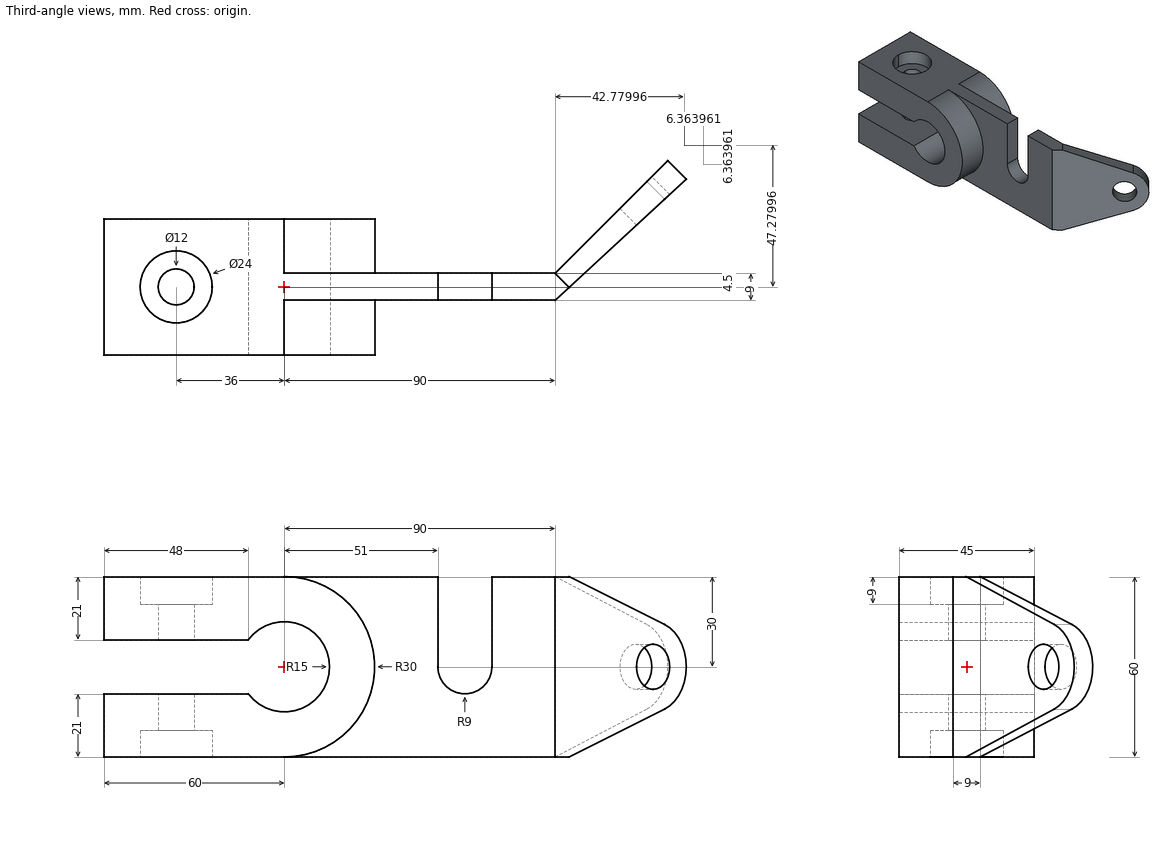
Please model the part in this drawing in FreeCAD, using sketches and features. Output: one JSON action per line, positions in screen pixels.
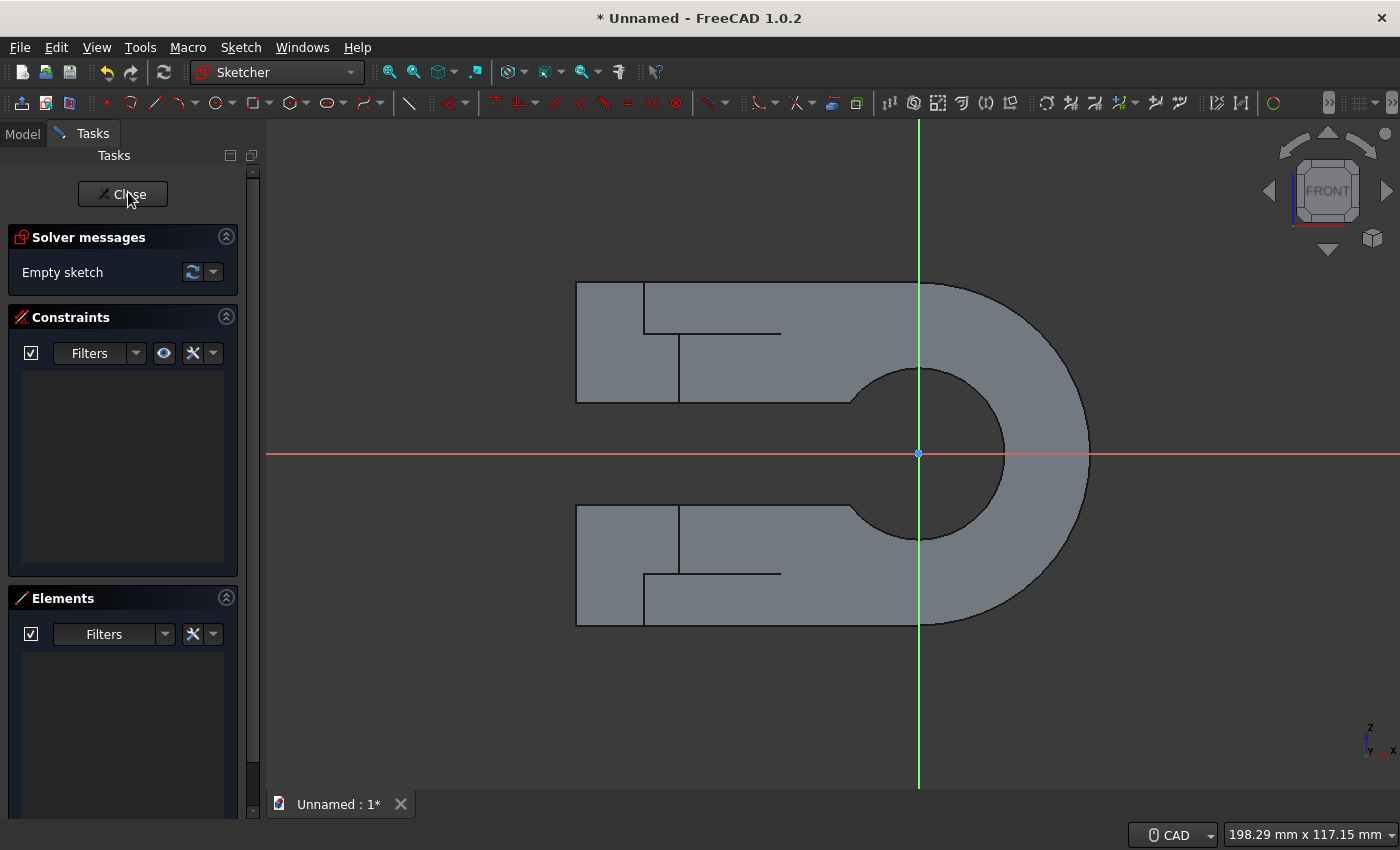
{"action": "scroll", "coordinate": [294, 454], "scroll_direction": "down", "scroll_amount": 2}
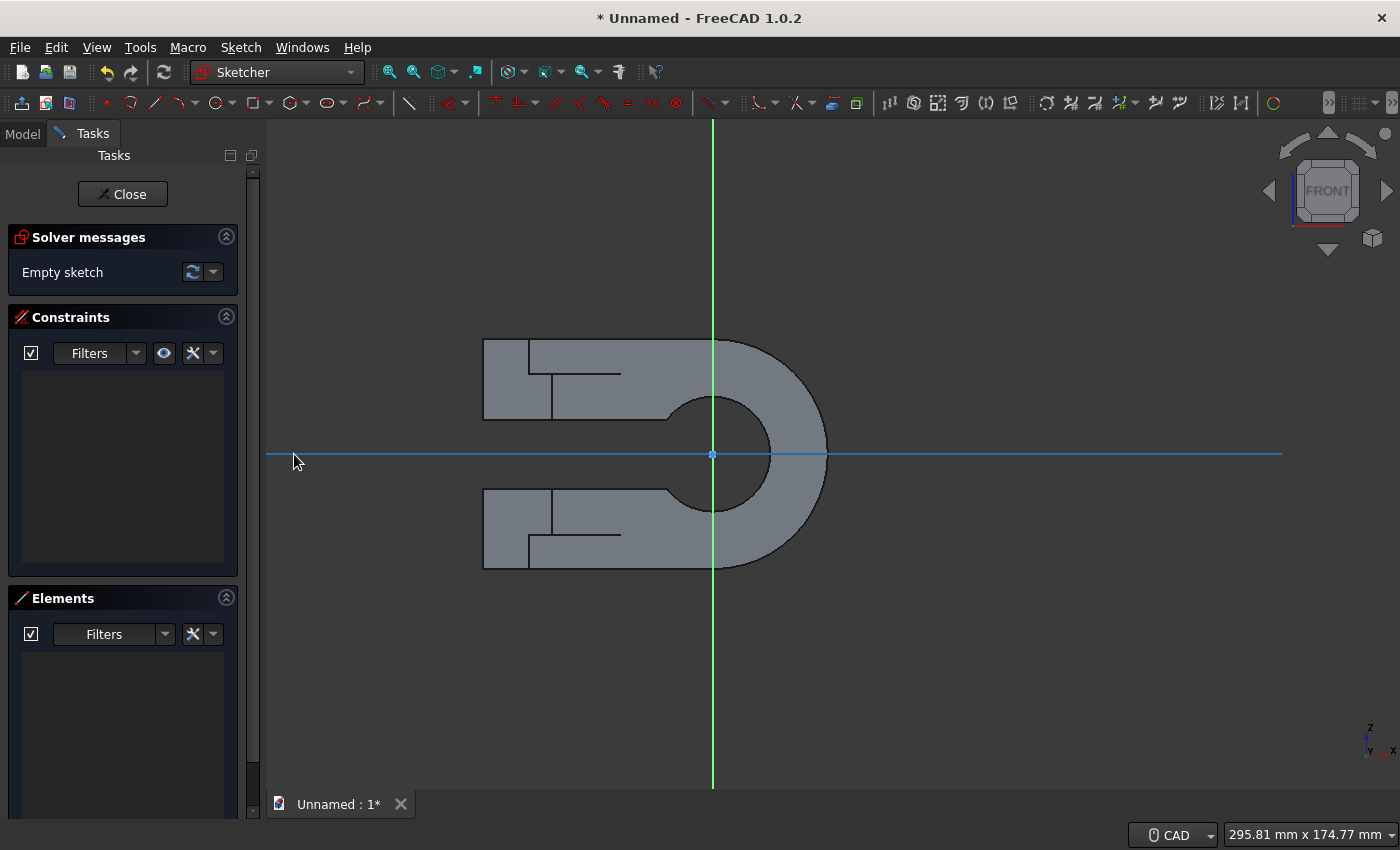
{"action": "scroll", "coordinate": [1032, 454], "scroll_direction": "up", "scroll_amount": 3}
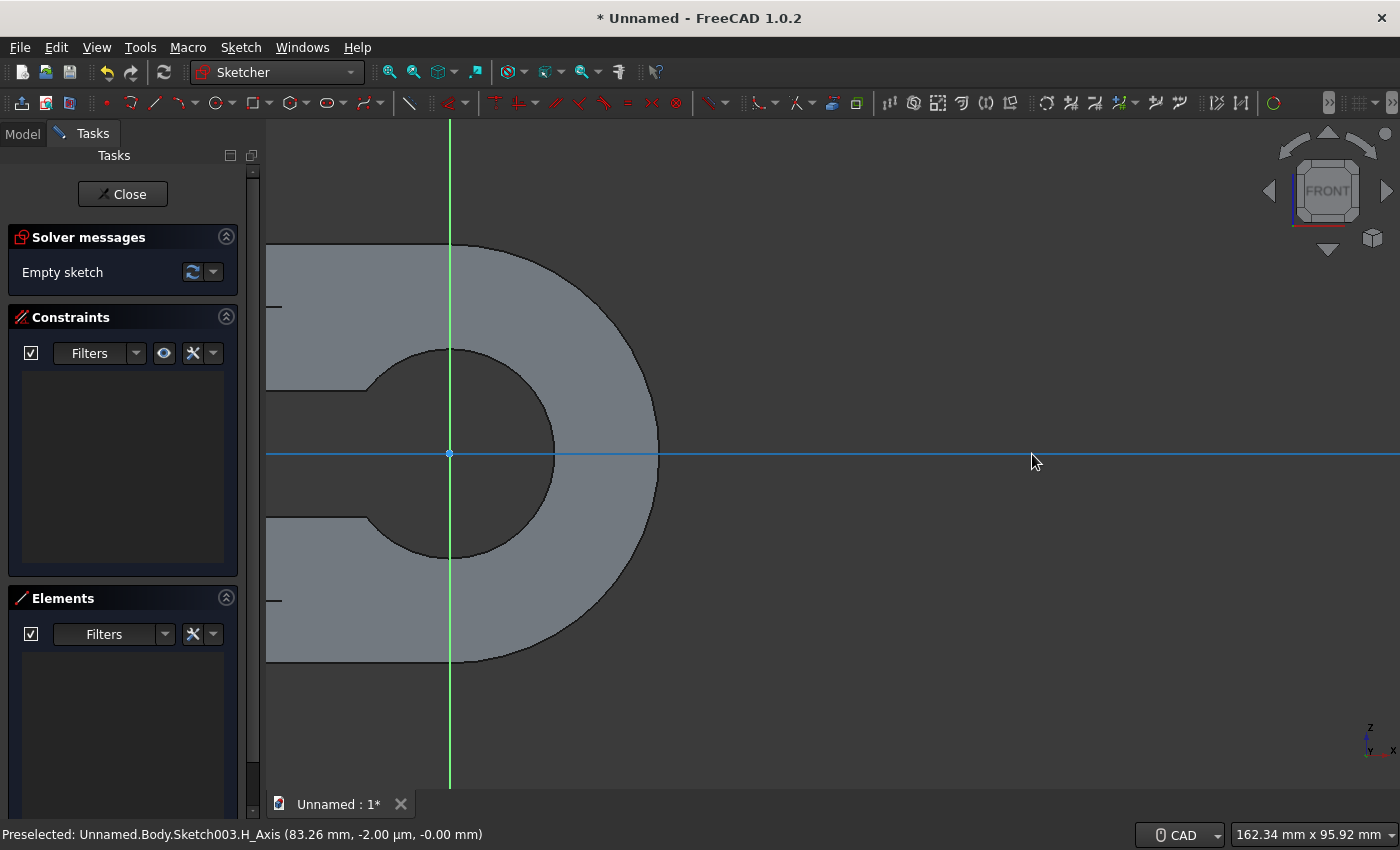
{"action": "key", "text": "g m"}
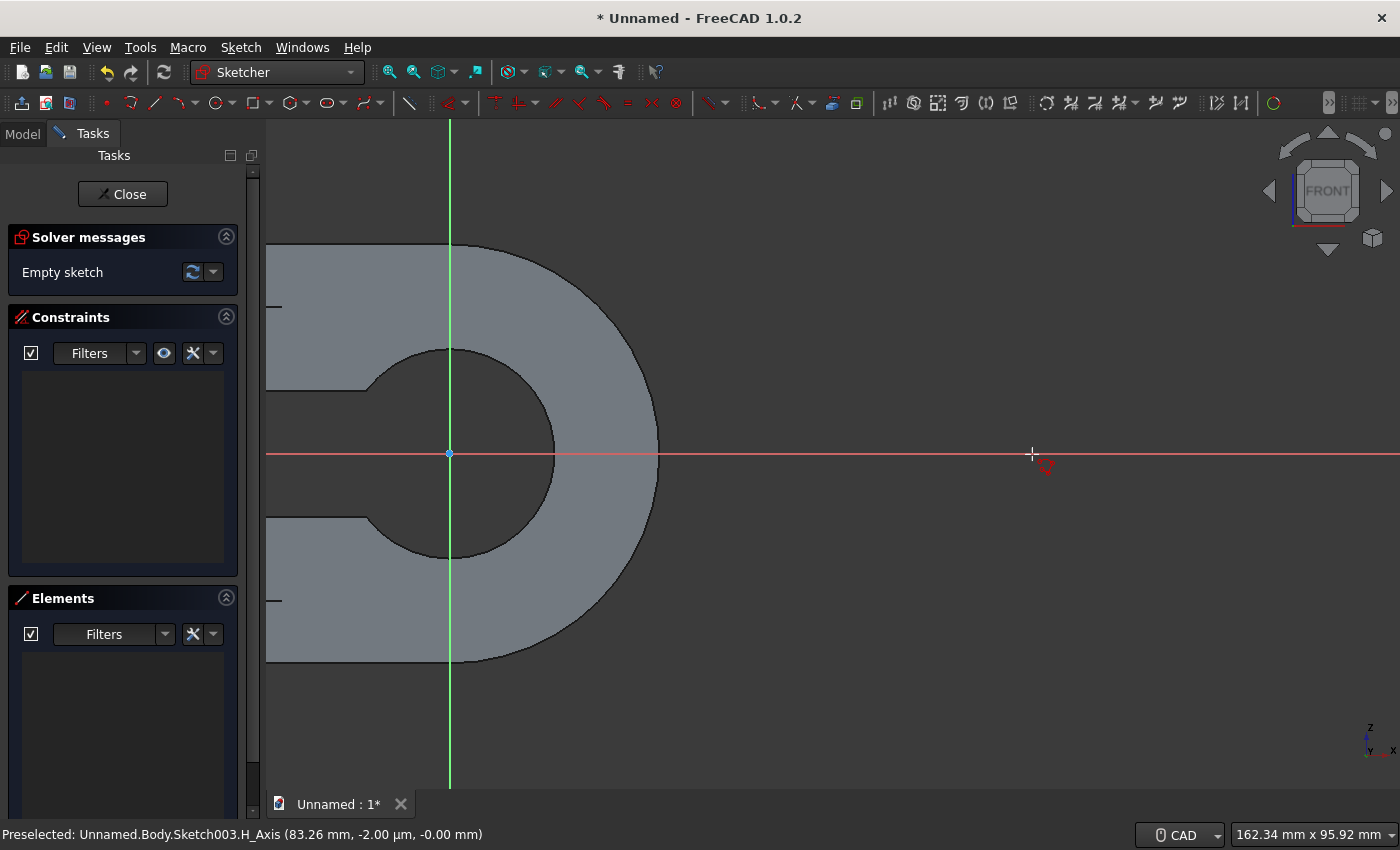
{"action": "left_click", "coordinate": [450, 244]}
{"action": "left_click", "coordinate": [1079, 244]}
{"action": "left_click", "coordinate": [1079, 663]}
{"action": "left_click", "coordinate": [450, 663]}
{"action": "right_click", "coordinate": [450, 663]}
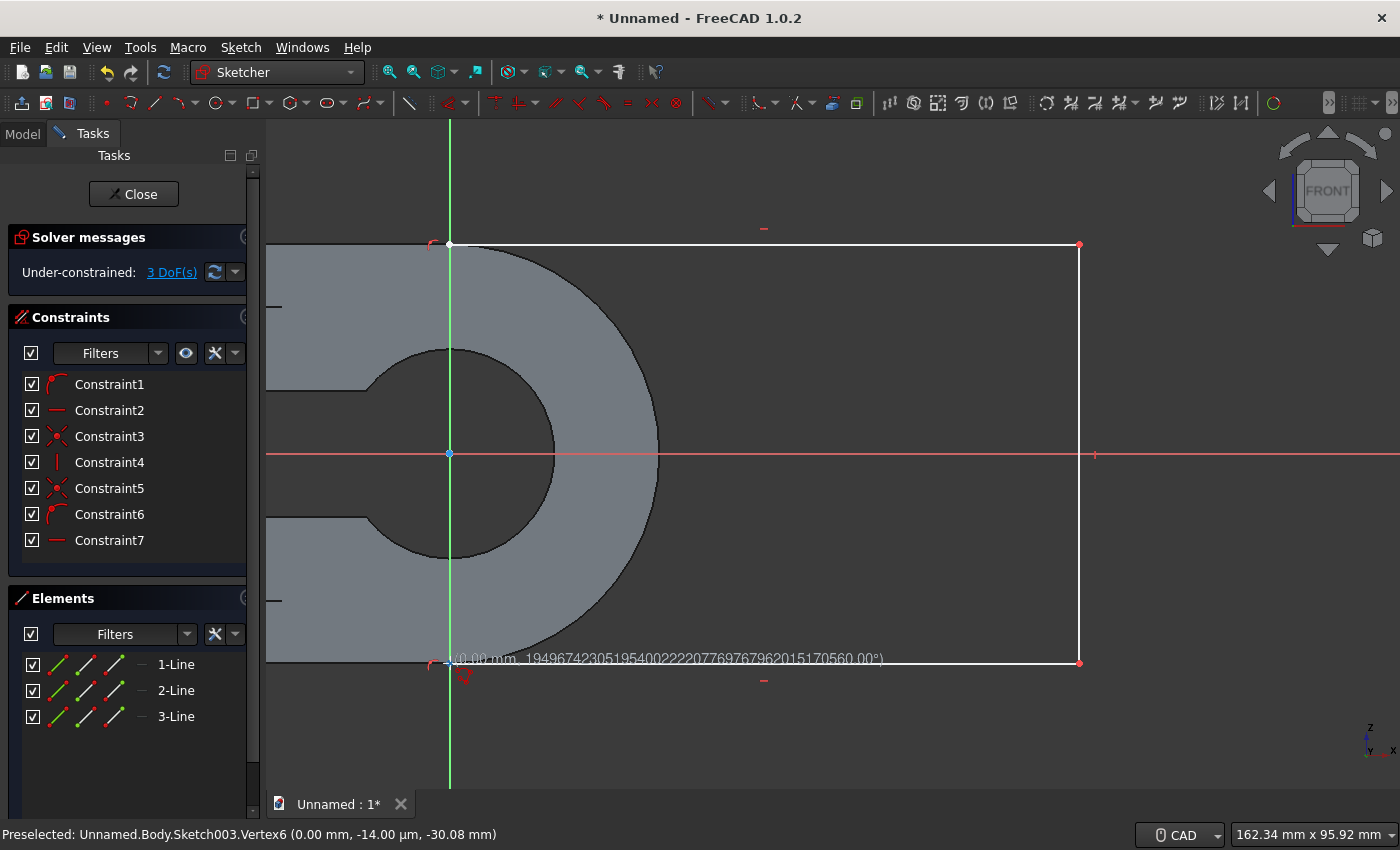
{"action": "key", "text": "g 3 a"}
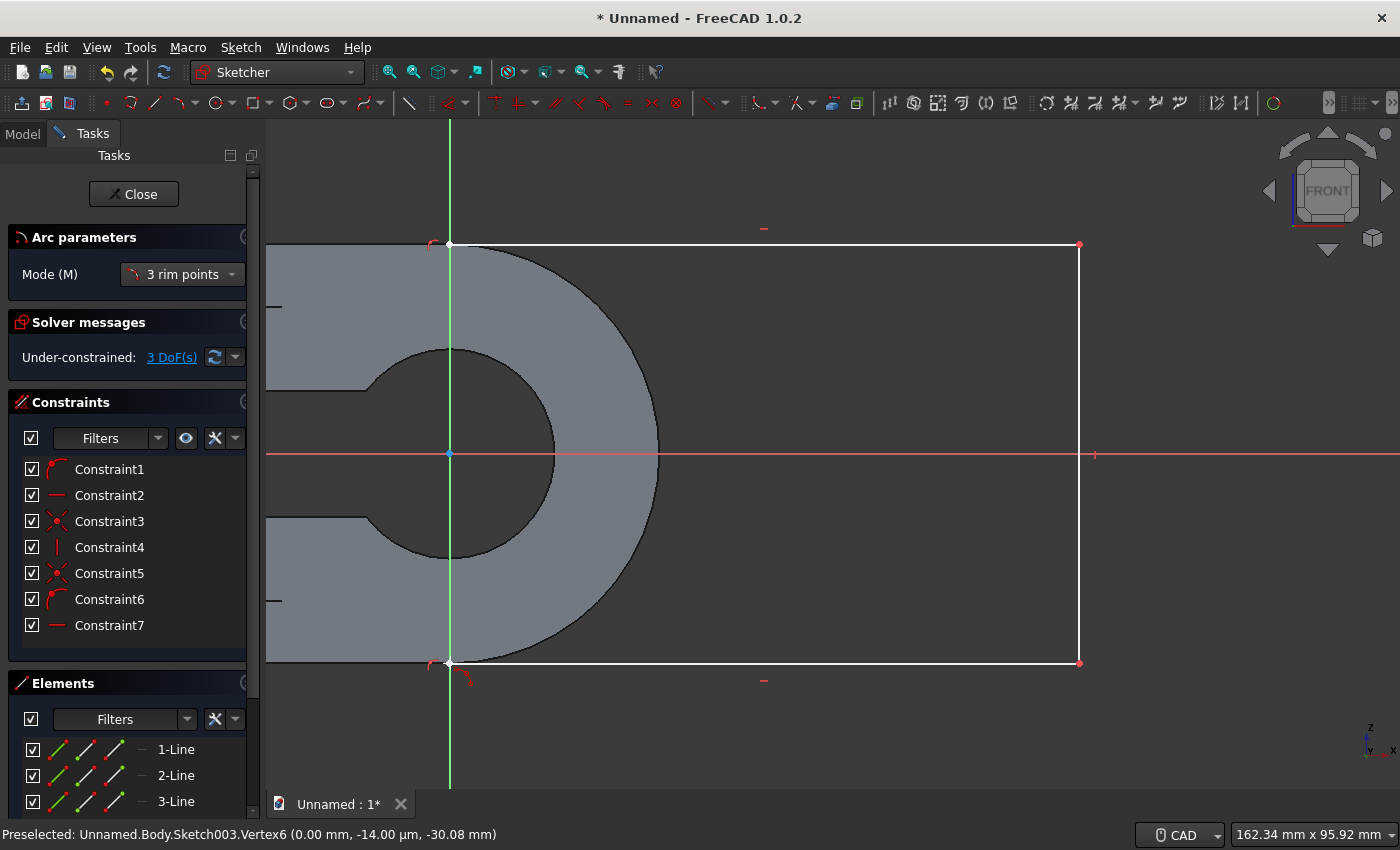
{"action": "left_click", "coordinate": [450, 664]}
{"action": "left_click", "coordinate": [450, 245]}
{"action": "left_click", "coordinate": [649, 519]}
{"action": "key", "text": "Escape"}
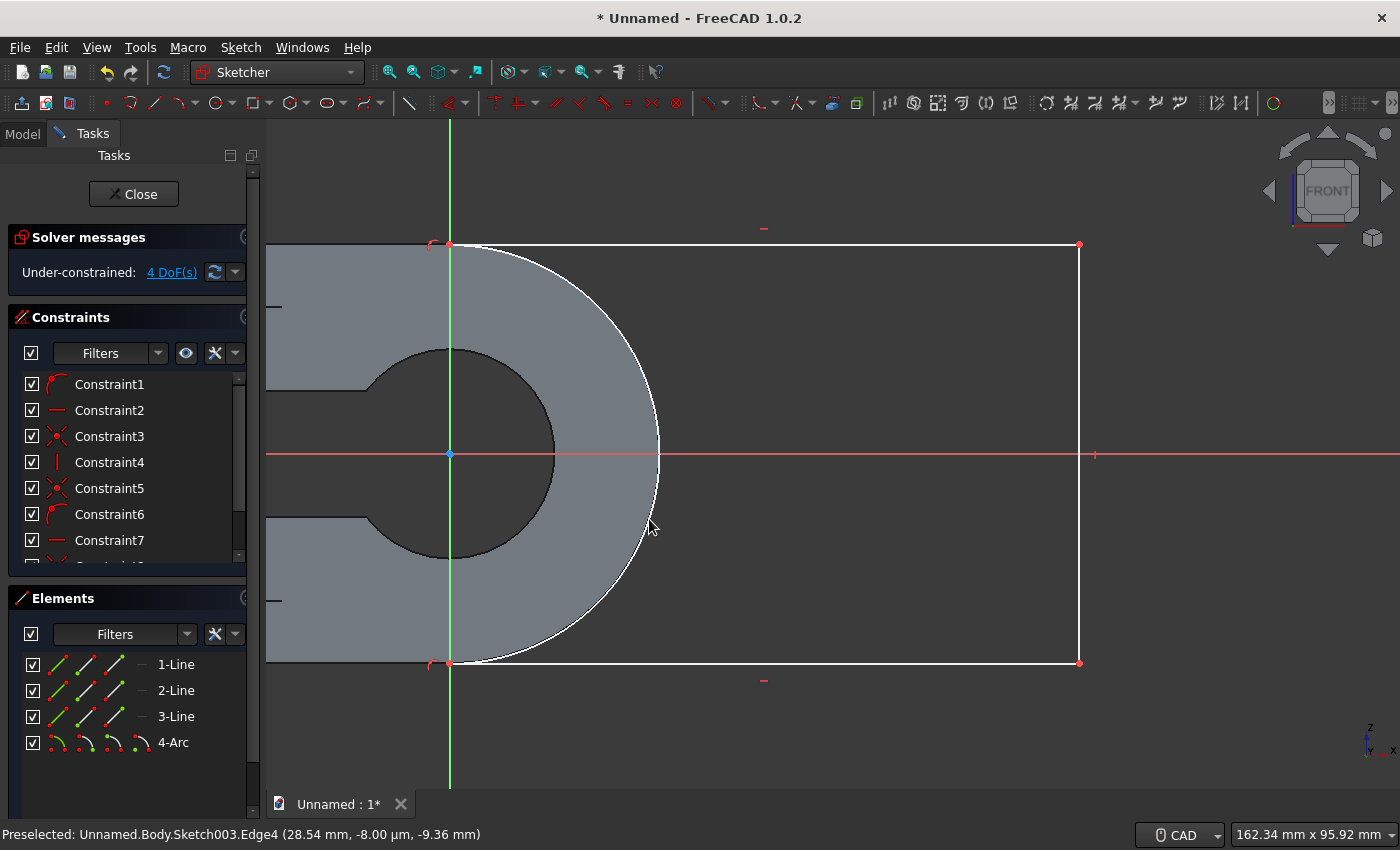
{"action": "left_click_drag", "start_coordinate": [440, 444], "coordinate": [460, 464]}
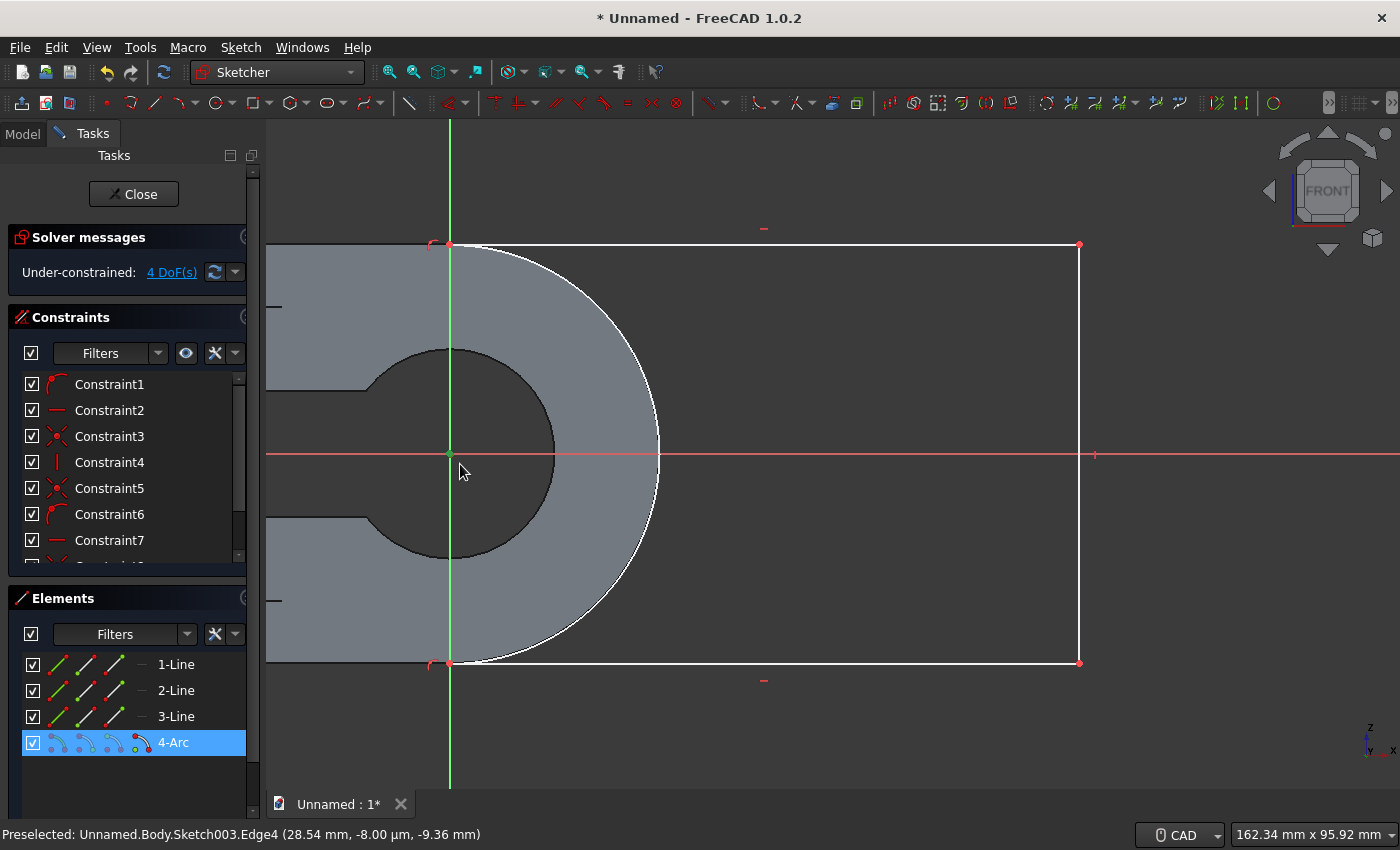
{"action": "key", "text": "c"}